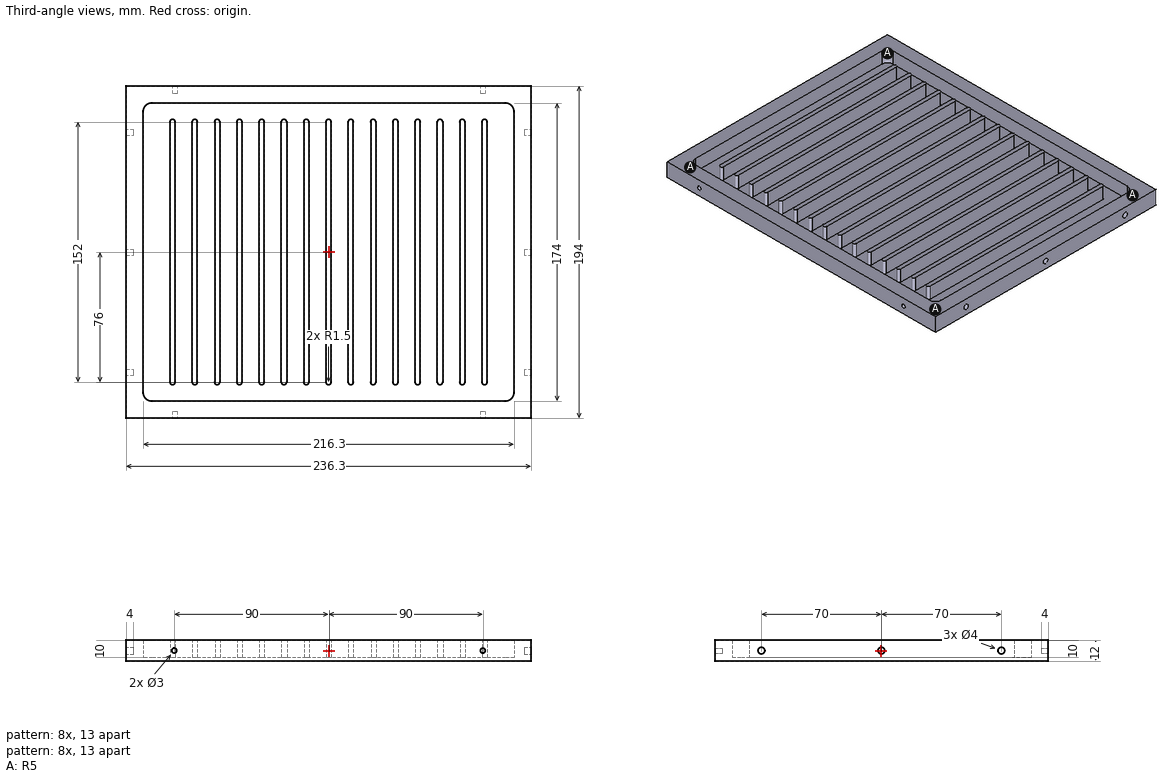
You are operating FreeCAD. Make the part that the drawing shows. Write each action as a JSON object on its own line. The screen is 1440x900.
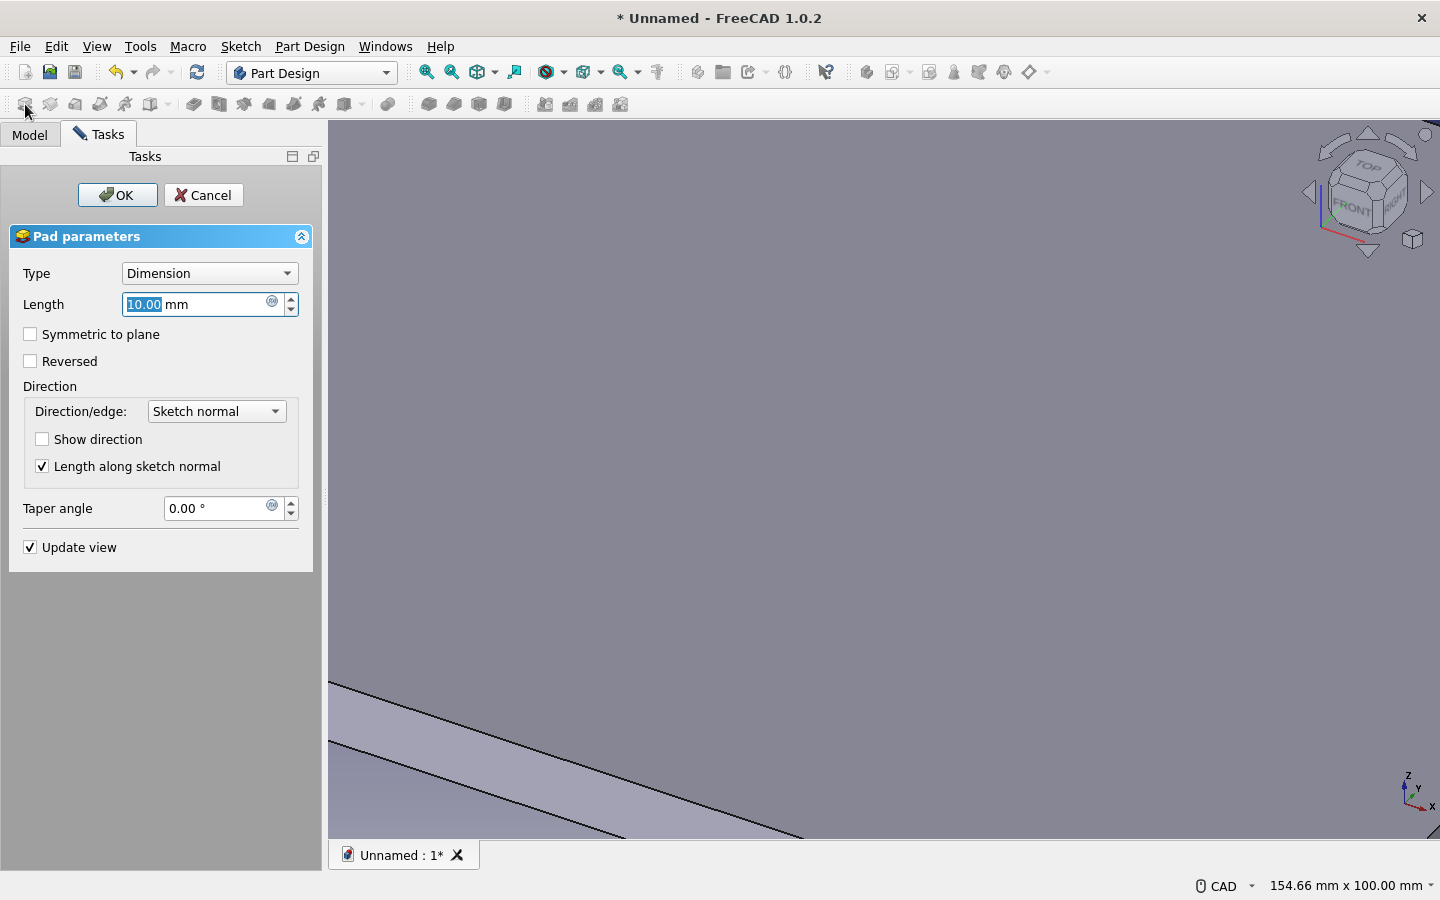
{"action": "type", "text": "12"}
{"action": "key", "text": "Tab"}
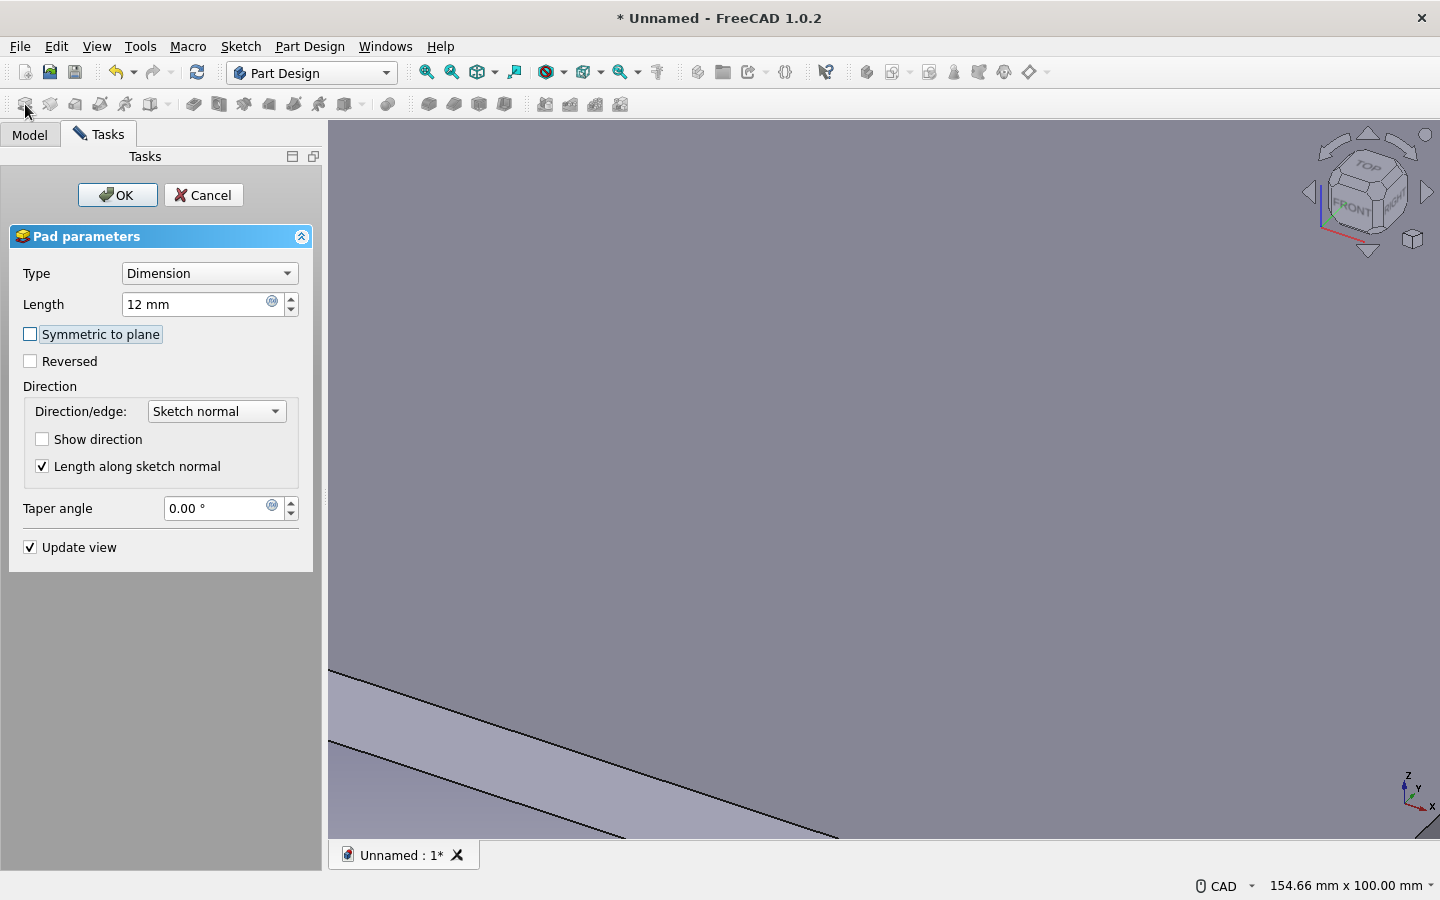
{"action": "left_click", "coordinate": [31, 334]}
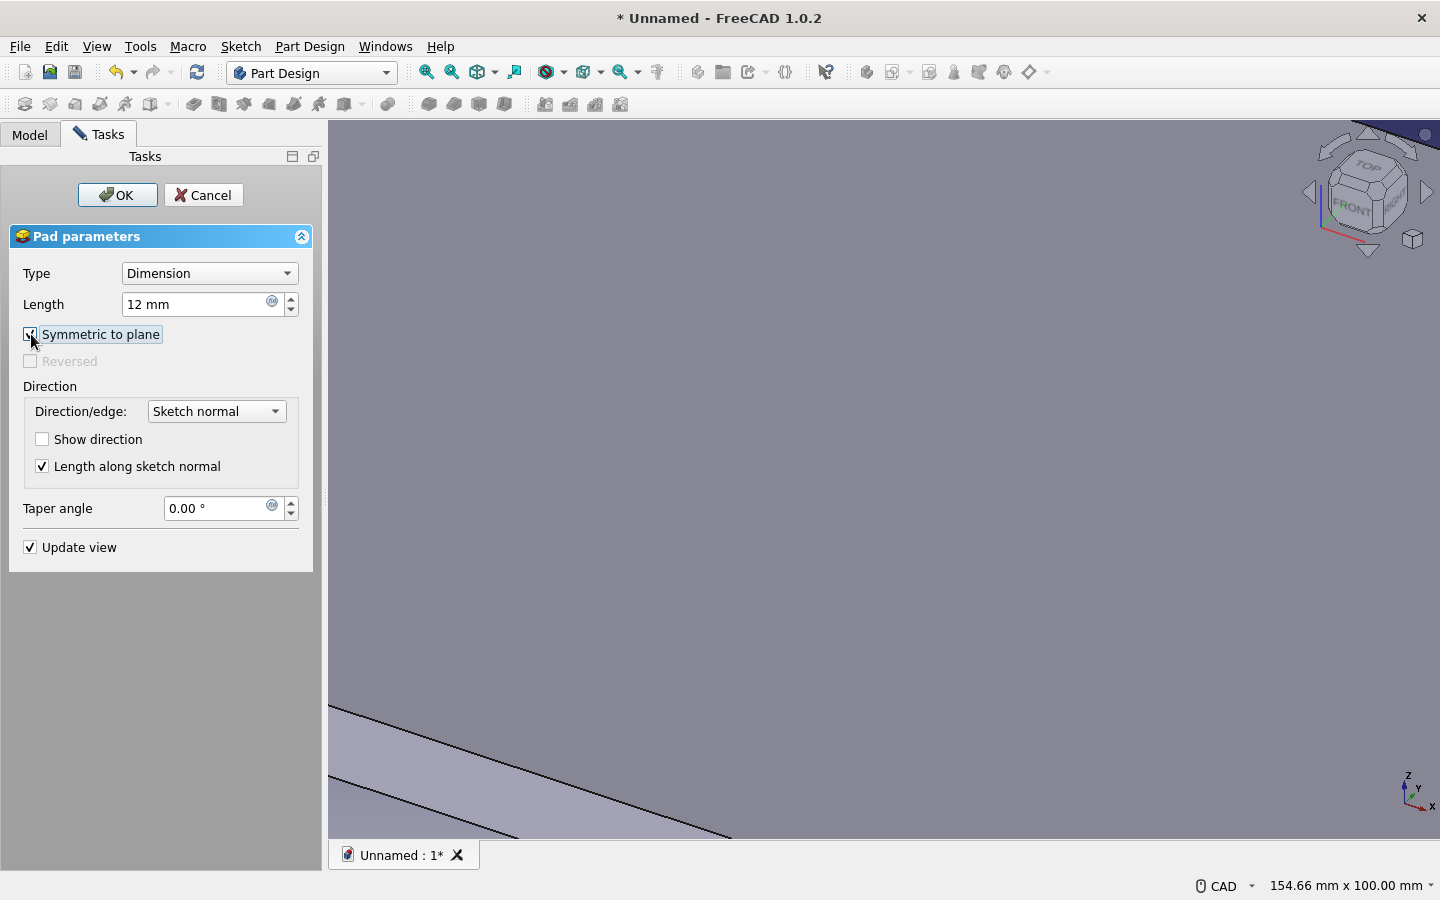
{"action": "left_click", "coordinate": [118, 195]}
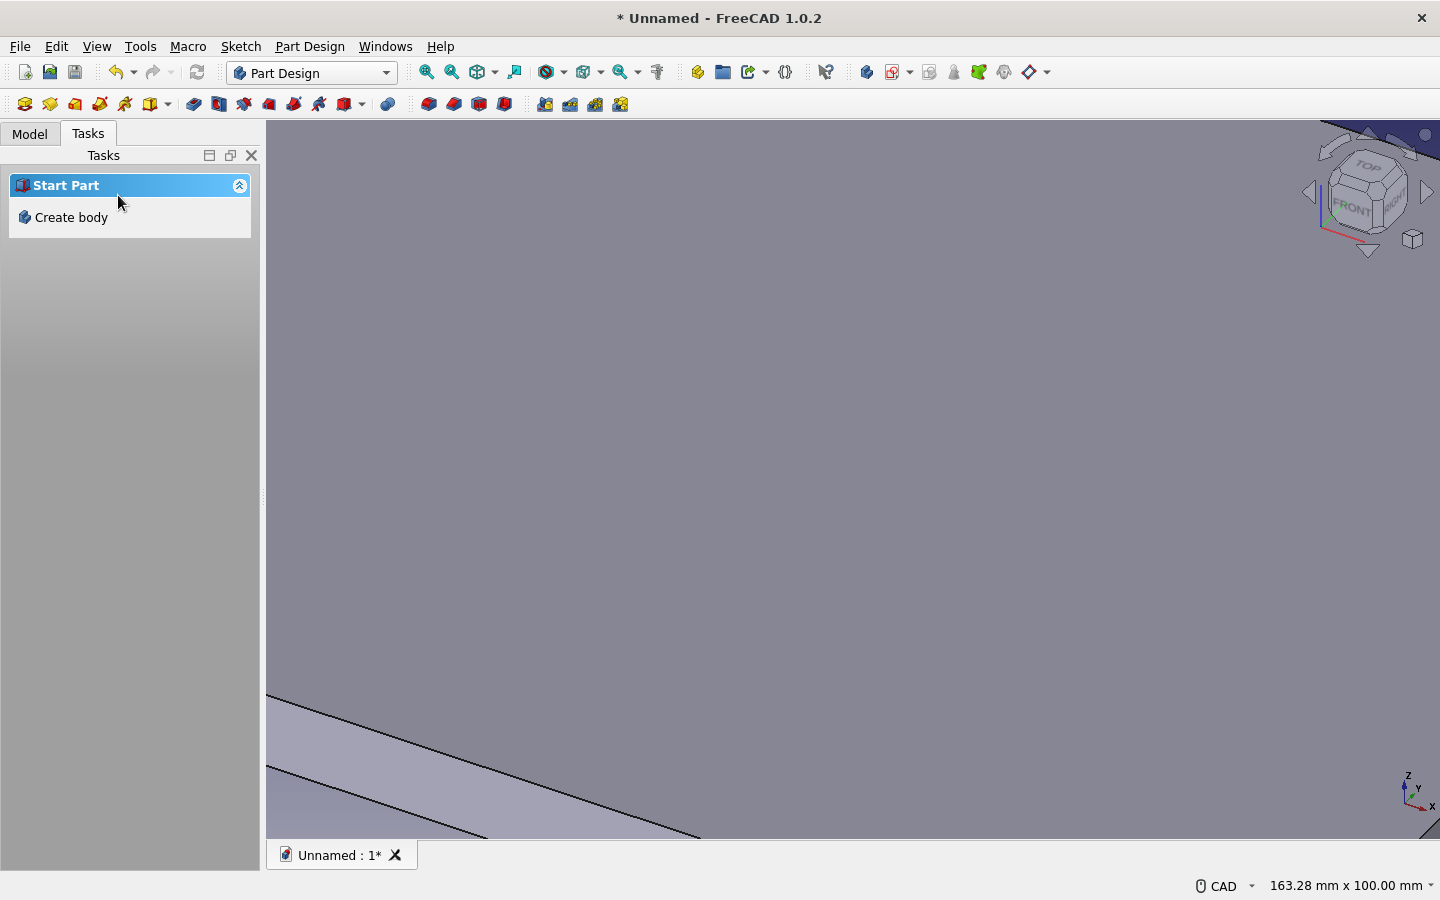
{"action": "left_click", "coordinate": [427, 72]}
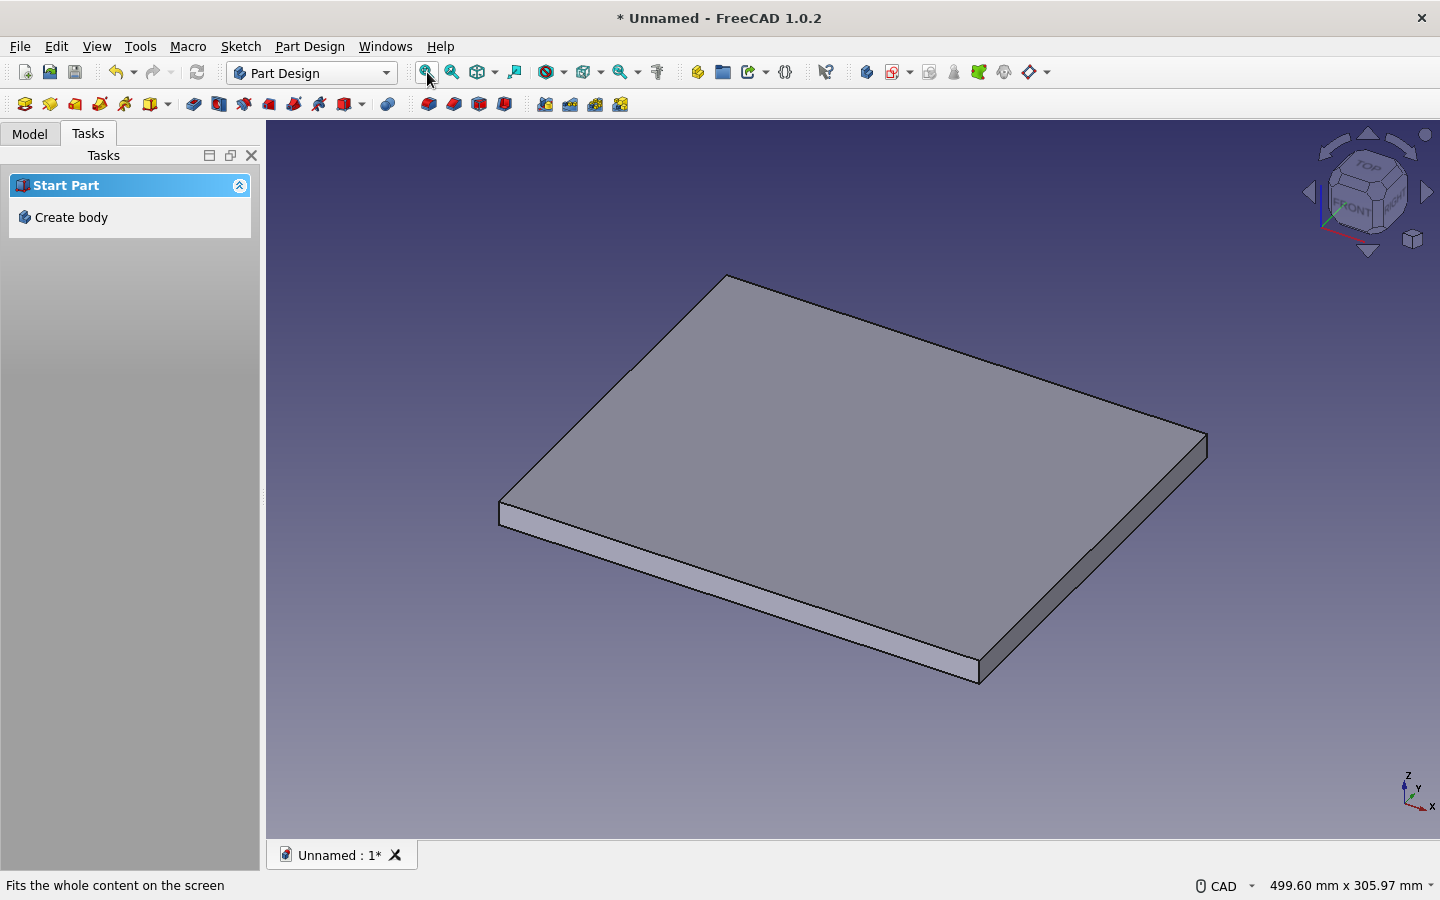
{"action": "left_click", "coordinate": [853, 467]}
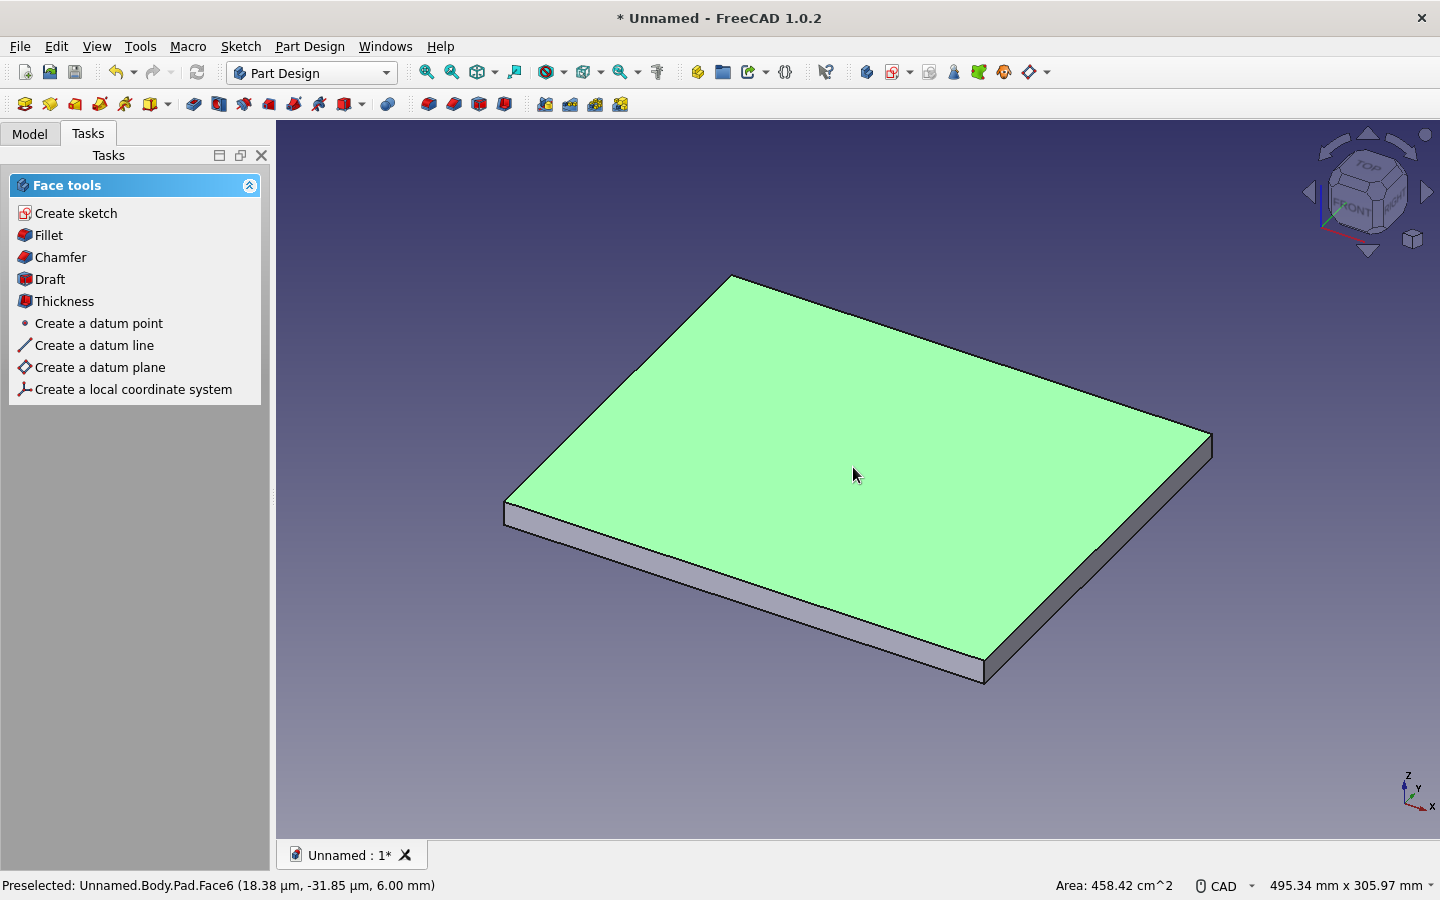
{"action": "left_click", "coordinate": [892, 72]}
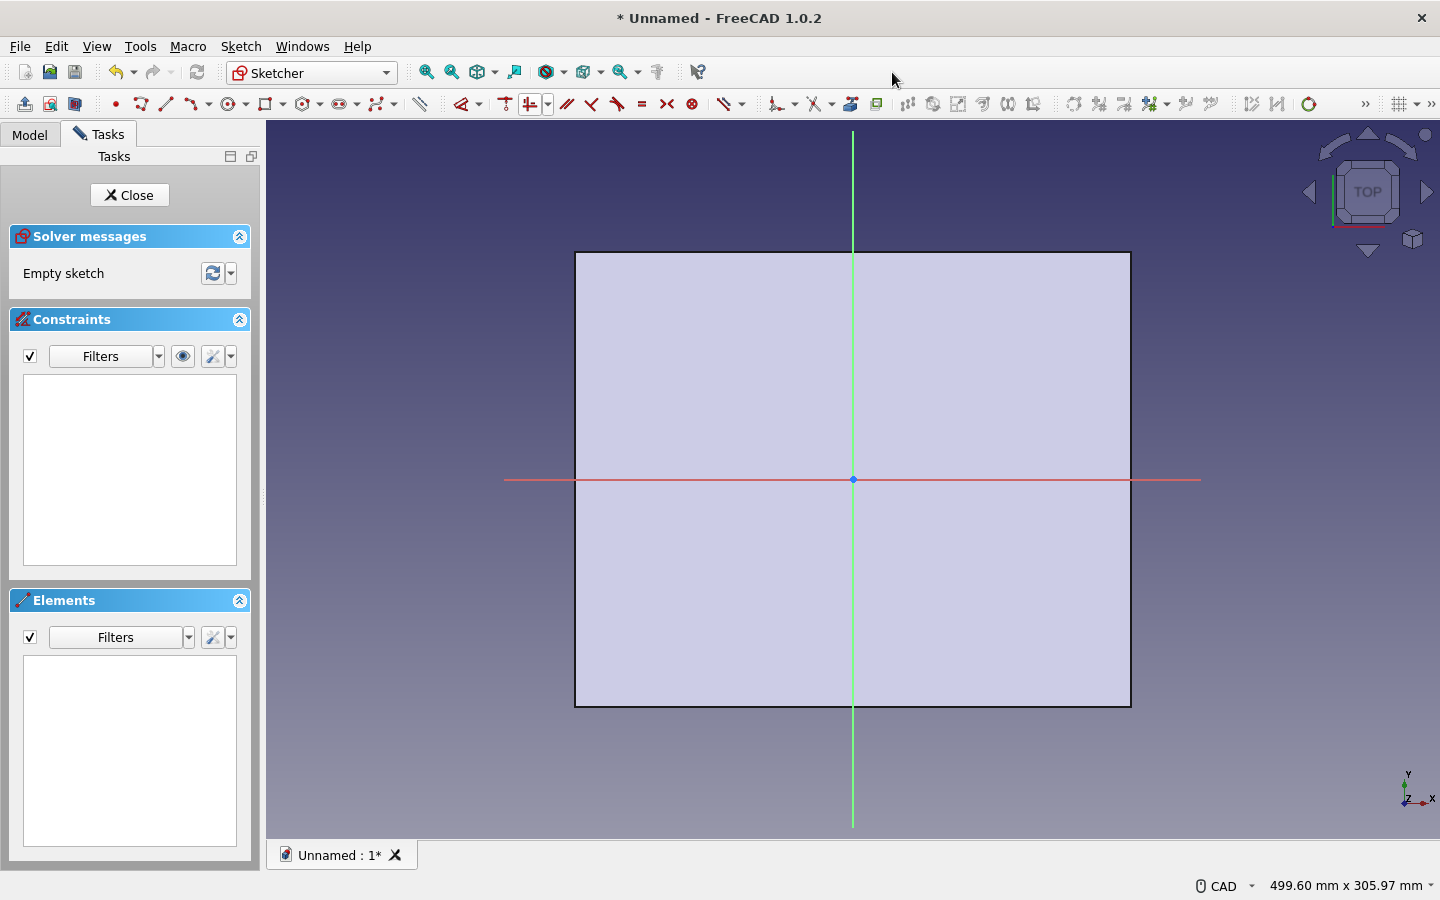
{"action": "key", "text": "g v"}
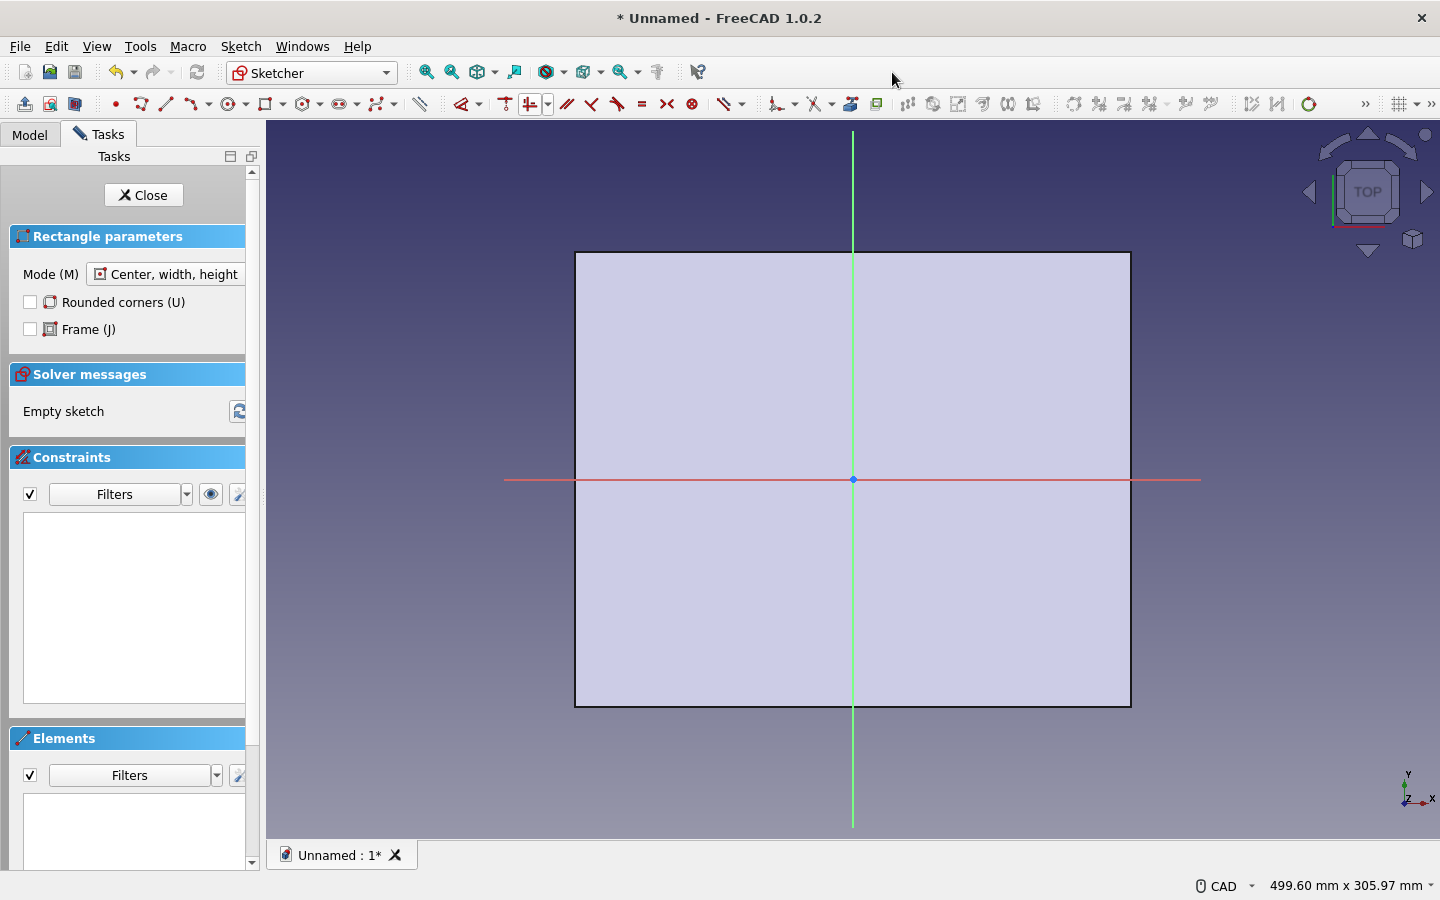
{"action": "left_click", "coordinate": [853, 480]}
{"action": "left_click", "coordinate": [1107, 275]}
{"action": "key", "text": "Escape"}